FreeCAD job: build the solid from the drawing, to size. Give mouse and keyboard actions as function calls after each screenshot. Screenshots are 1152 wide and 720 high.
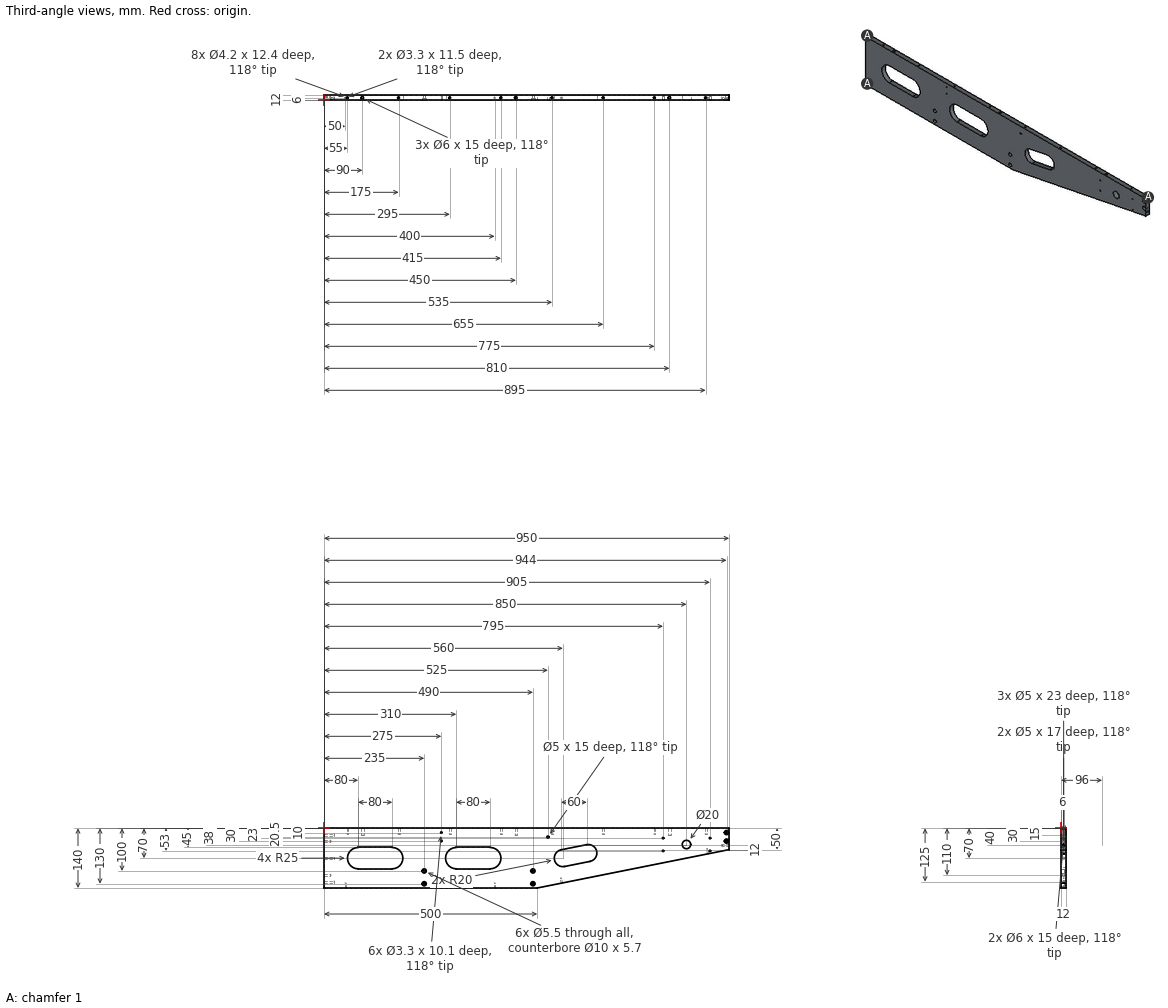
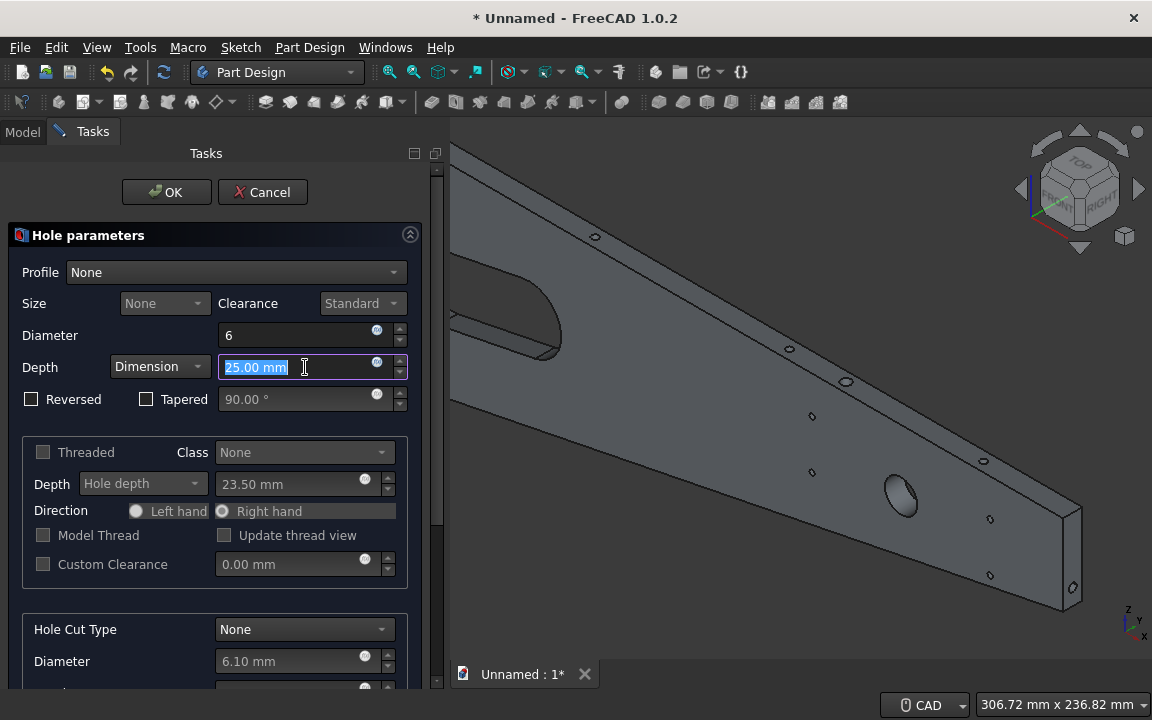
text(15)
key(Tab)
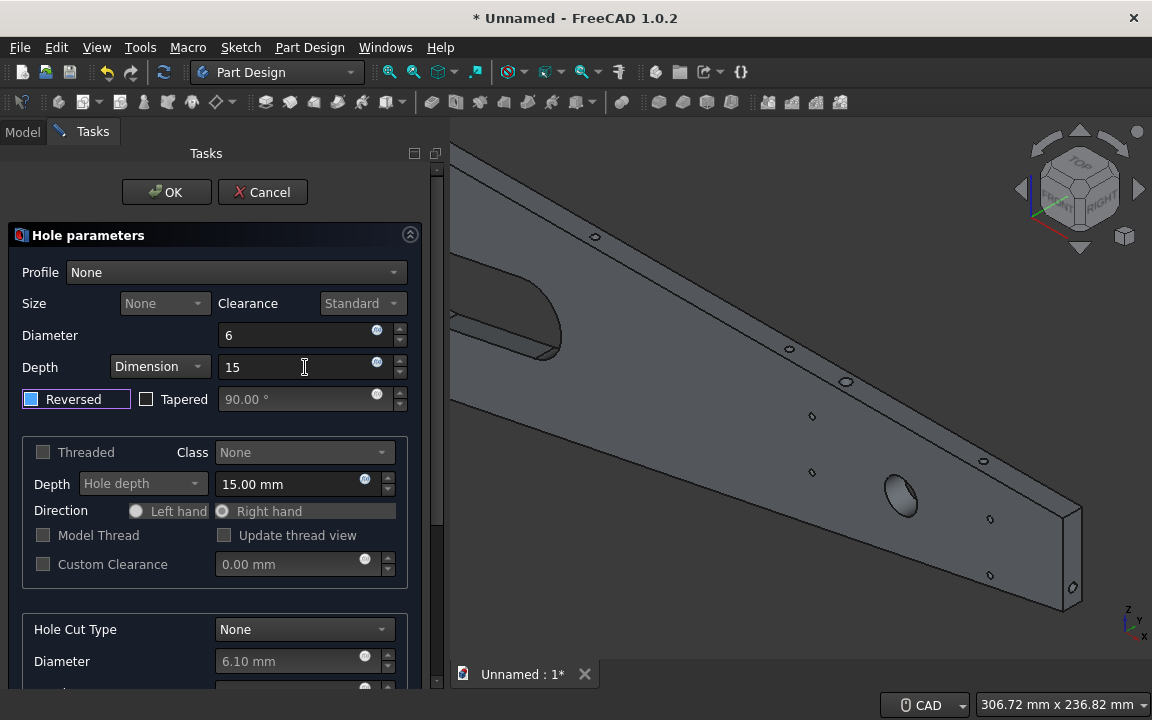
click(167, 192)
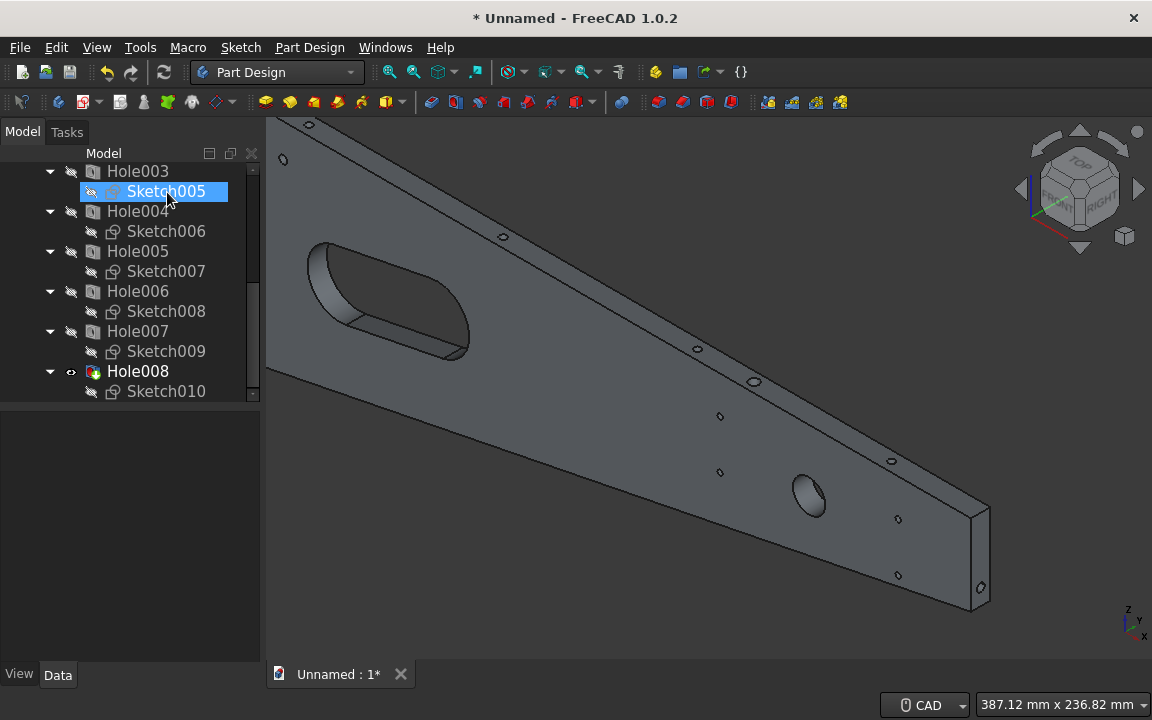
key(v)
key(f)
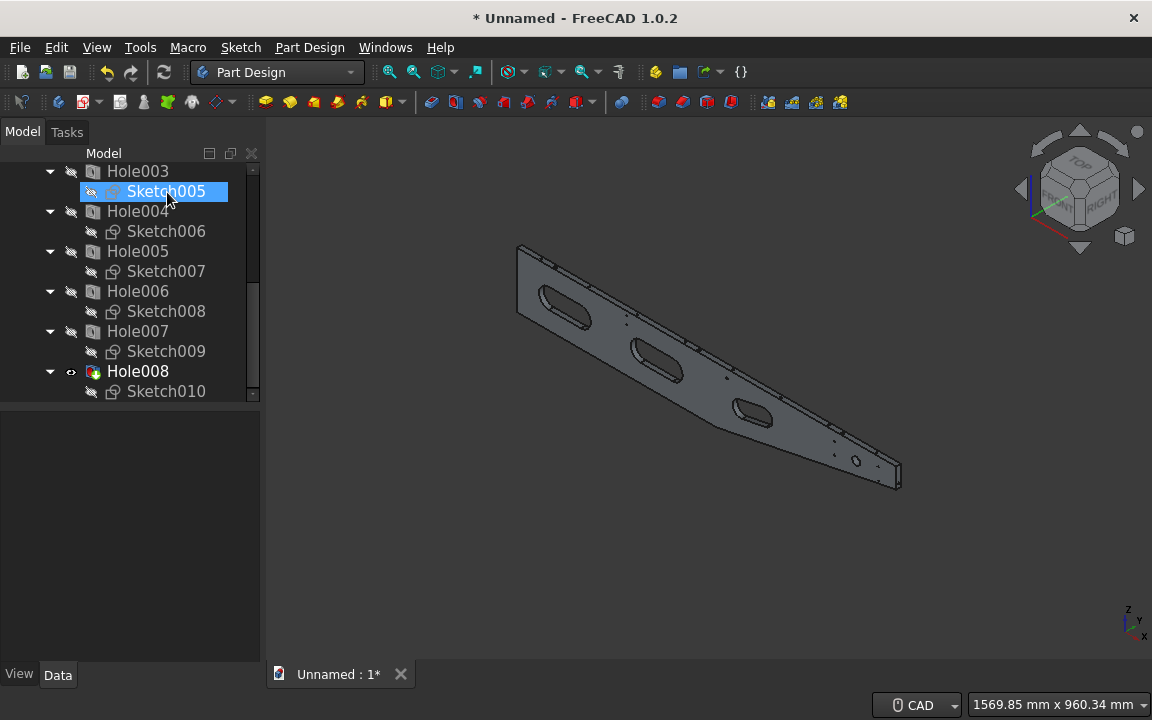
click(707, 388)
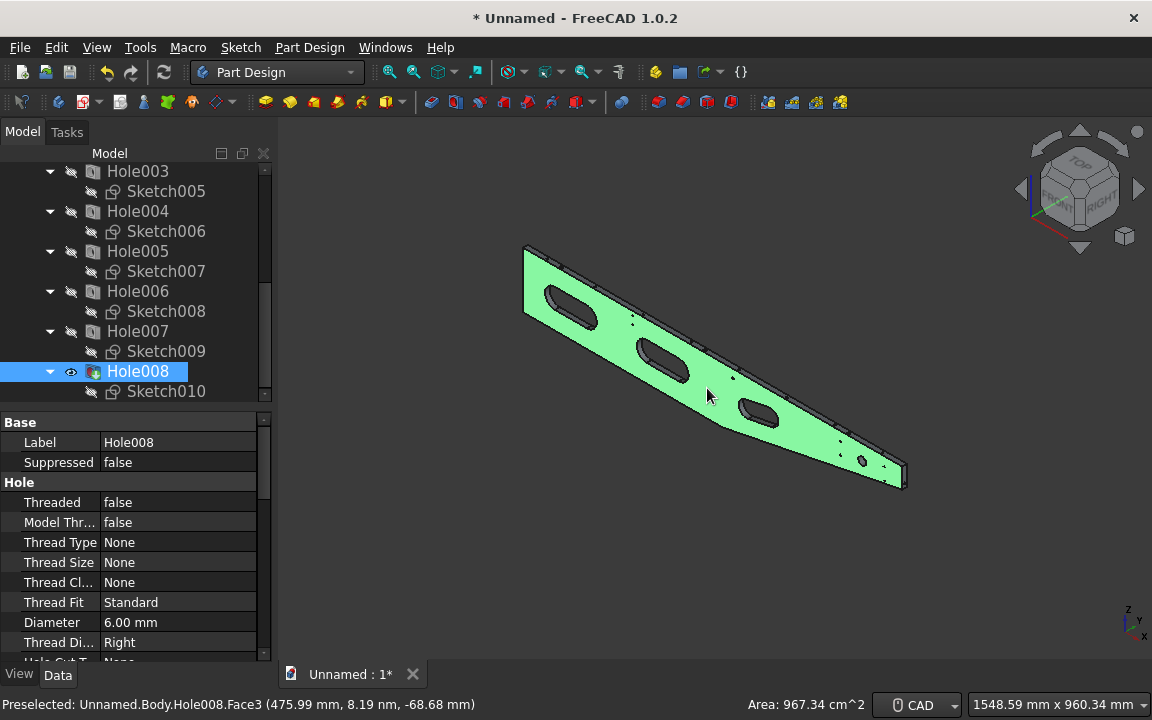
click(84, 102)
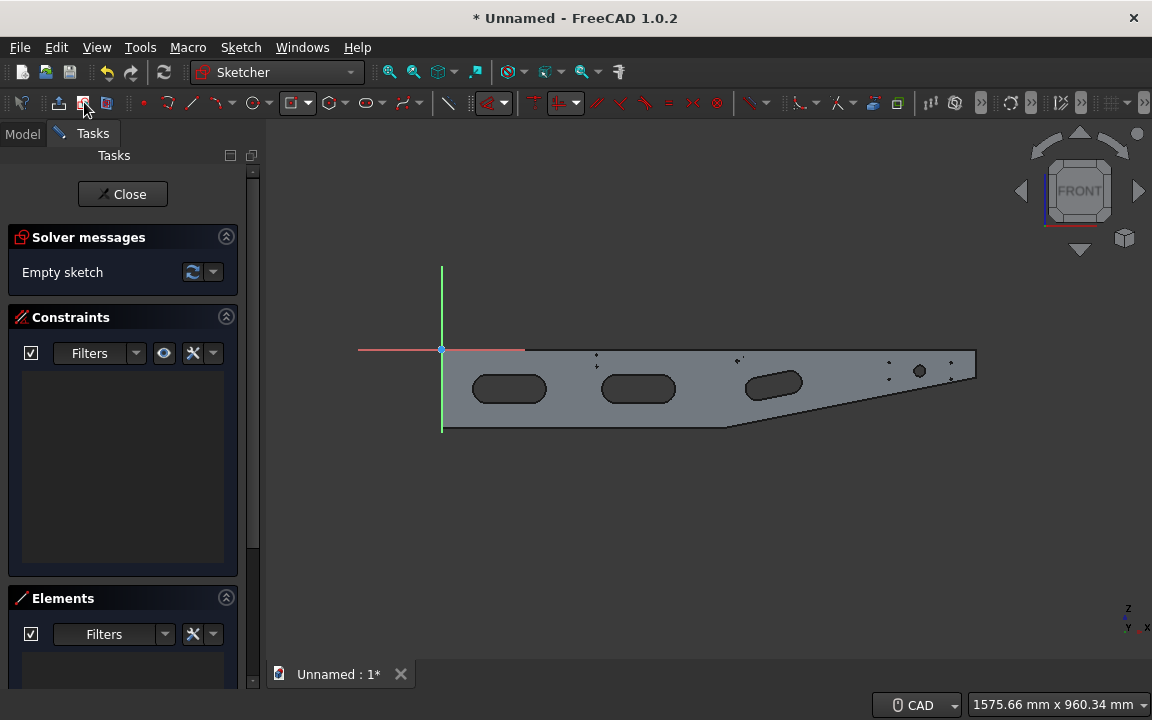
scroll(335, 398, down, 1)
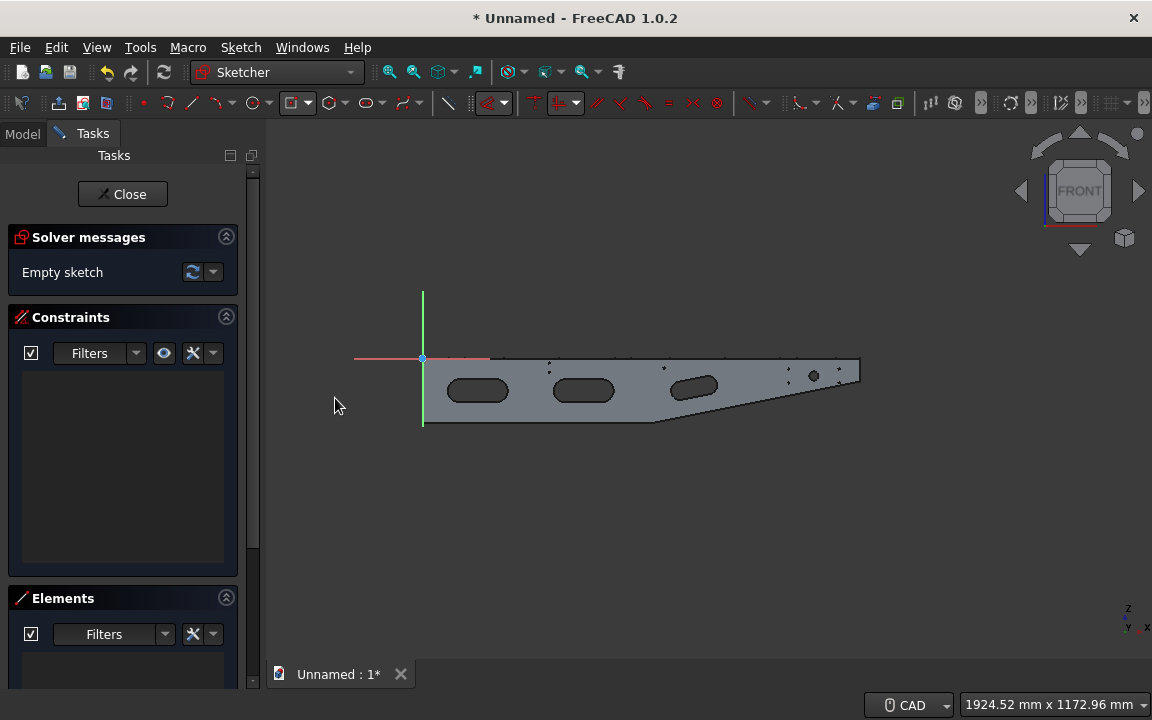
key(g)
key(c)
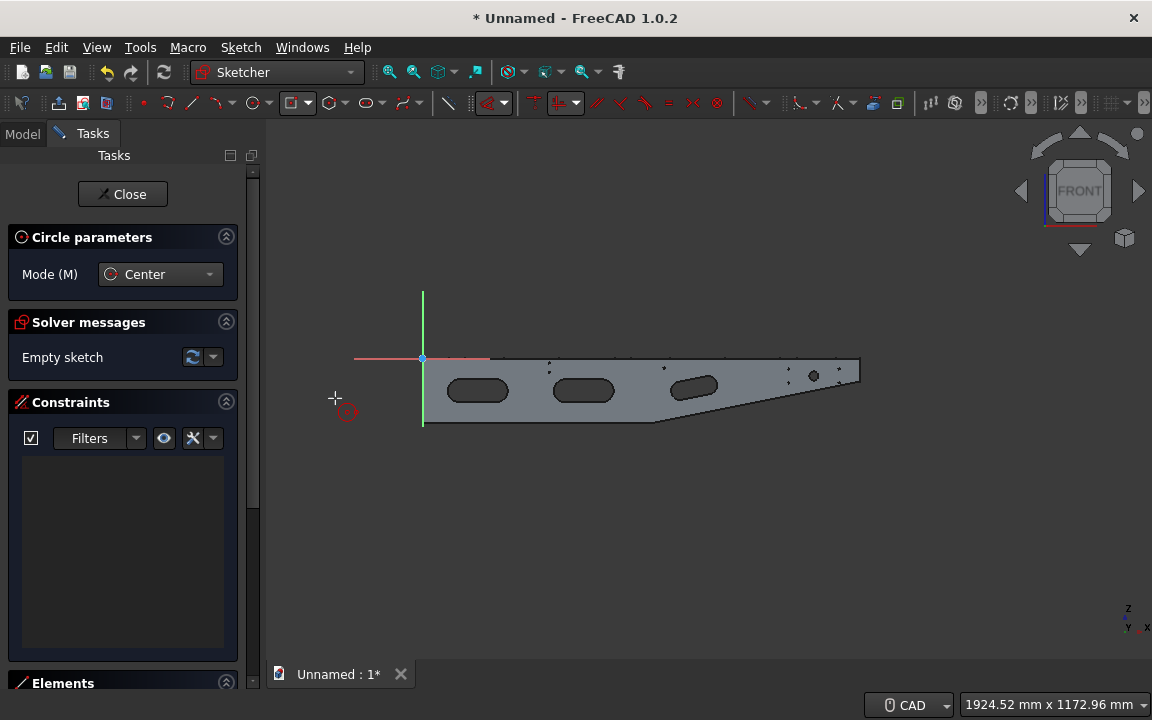
scroll(531, 405, up, 15)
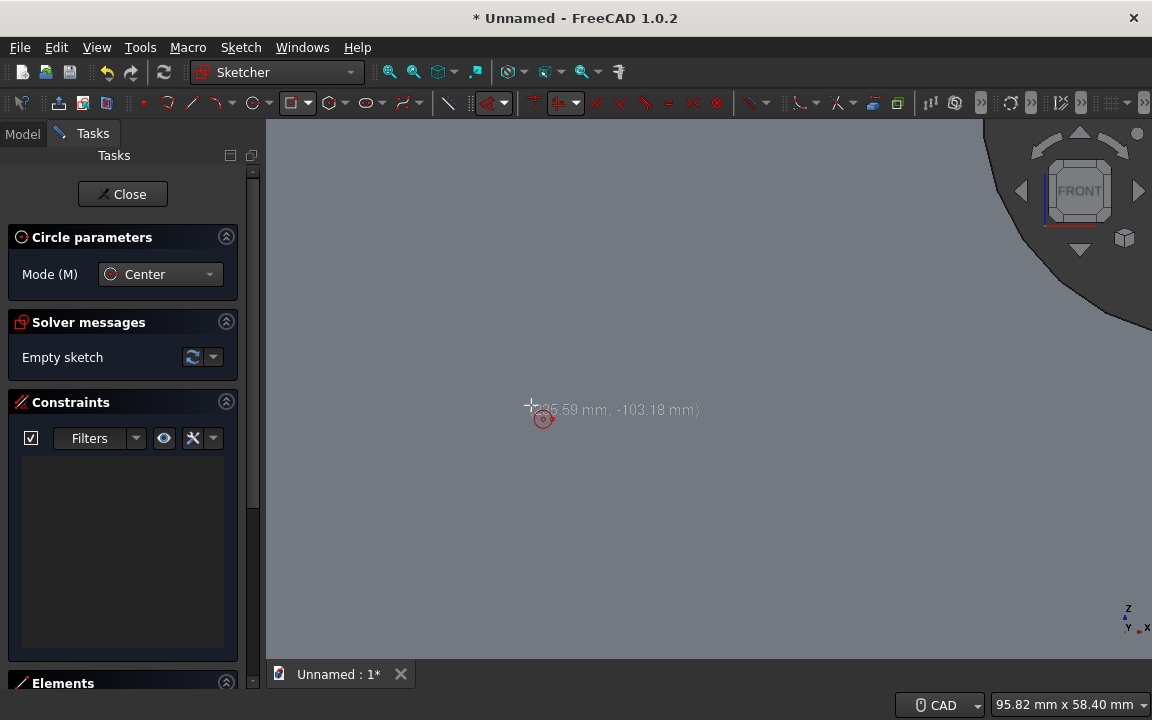
scroll(506, 409, down, 14)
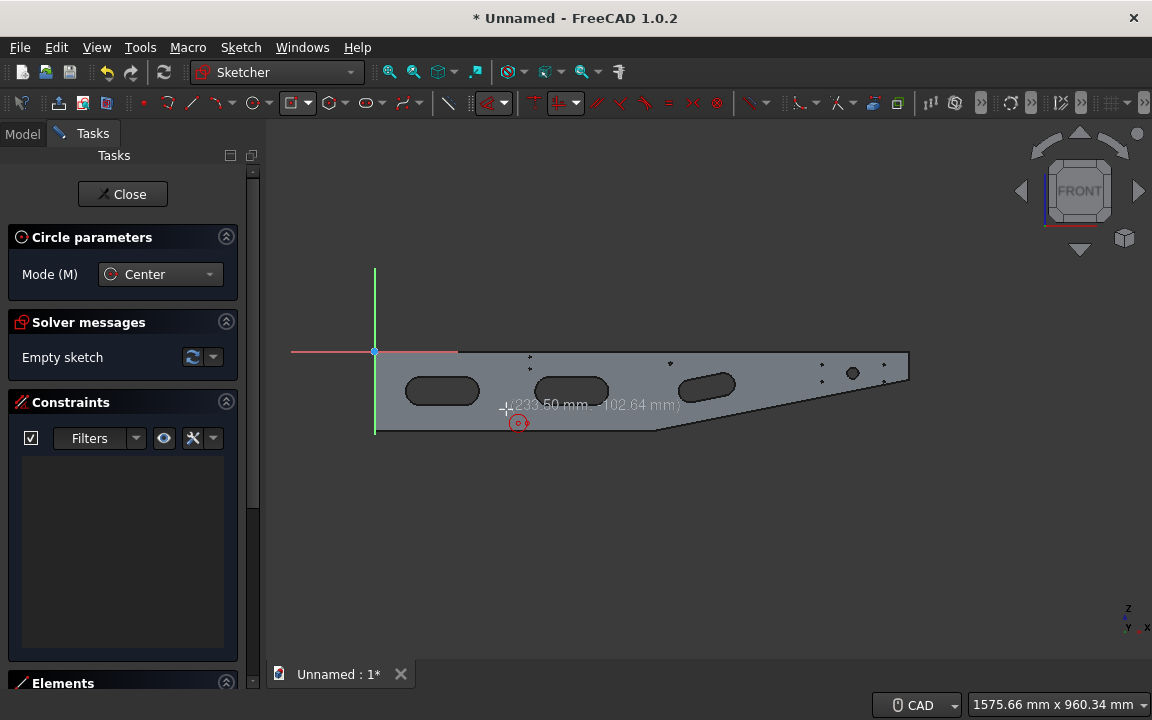
click(507, 408)
move(508, 407)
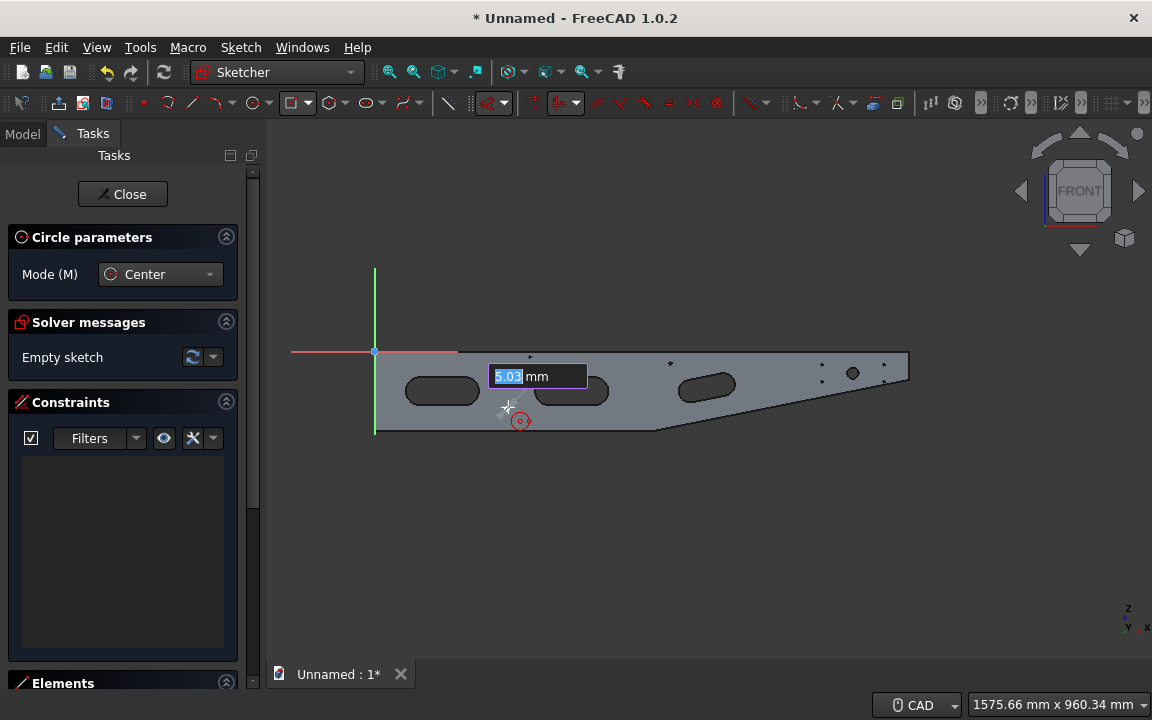
text(5.5)
key(Return)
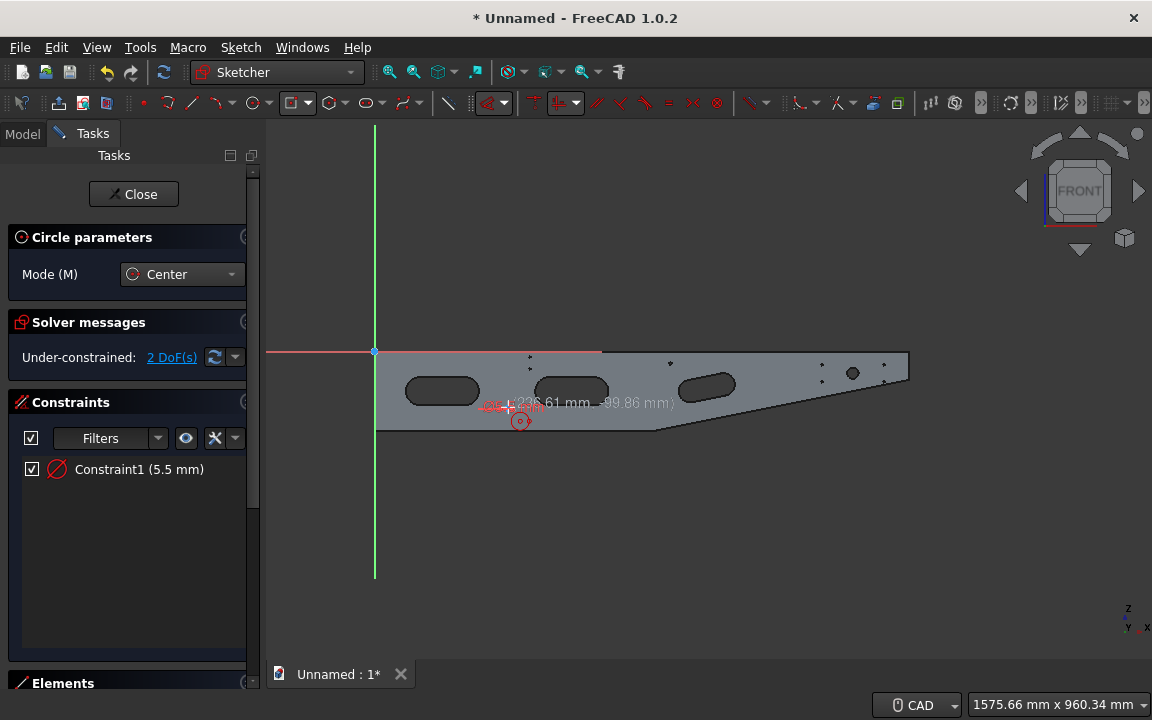
scroll(507, 425, up, 14)